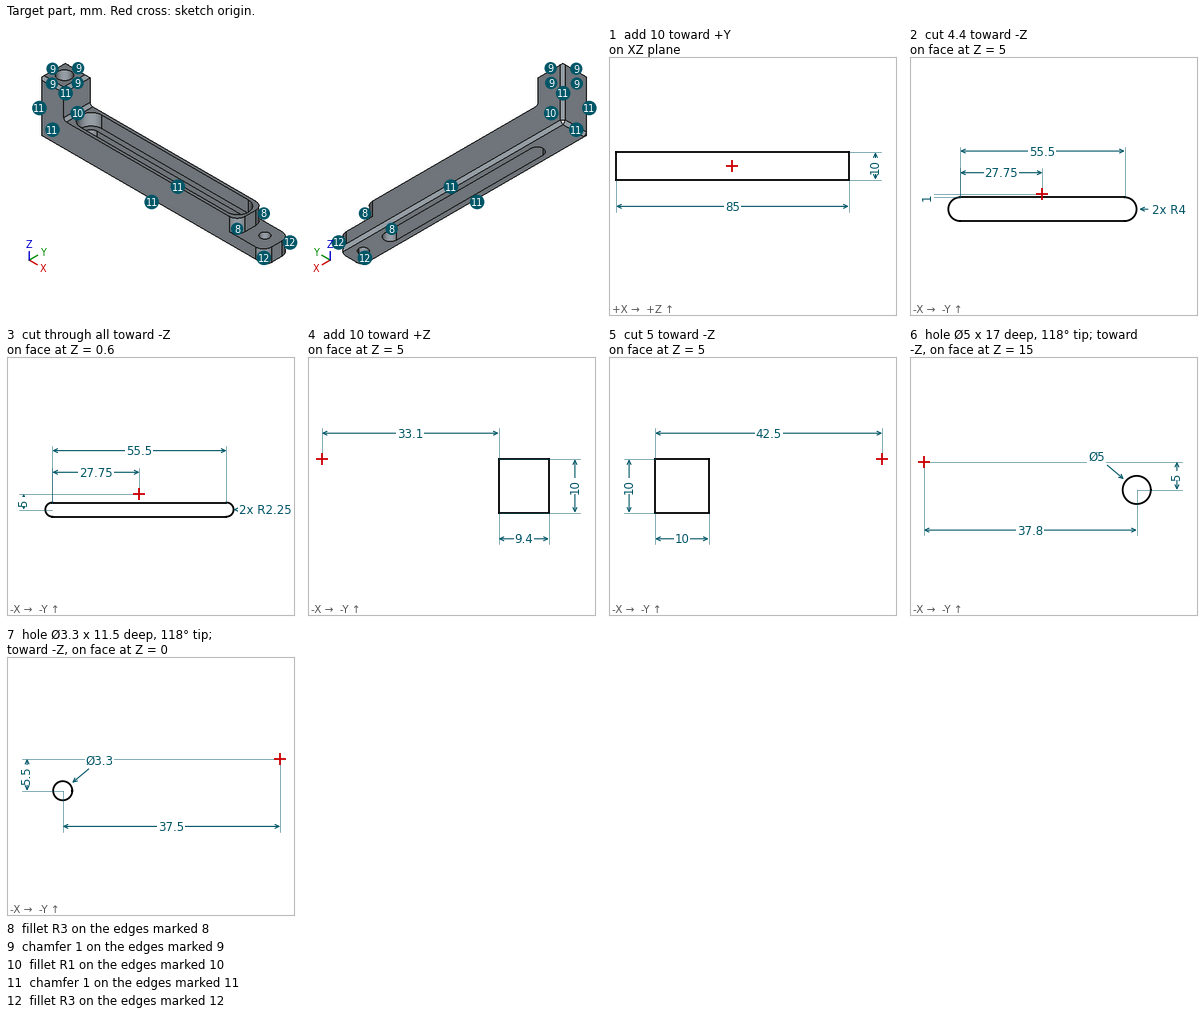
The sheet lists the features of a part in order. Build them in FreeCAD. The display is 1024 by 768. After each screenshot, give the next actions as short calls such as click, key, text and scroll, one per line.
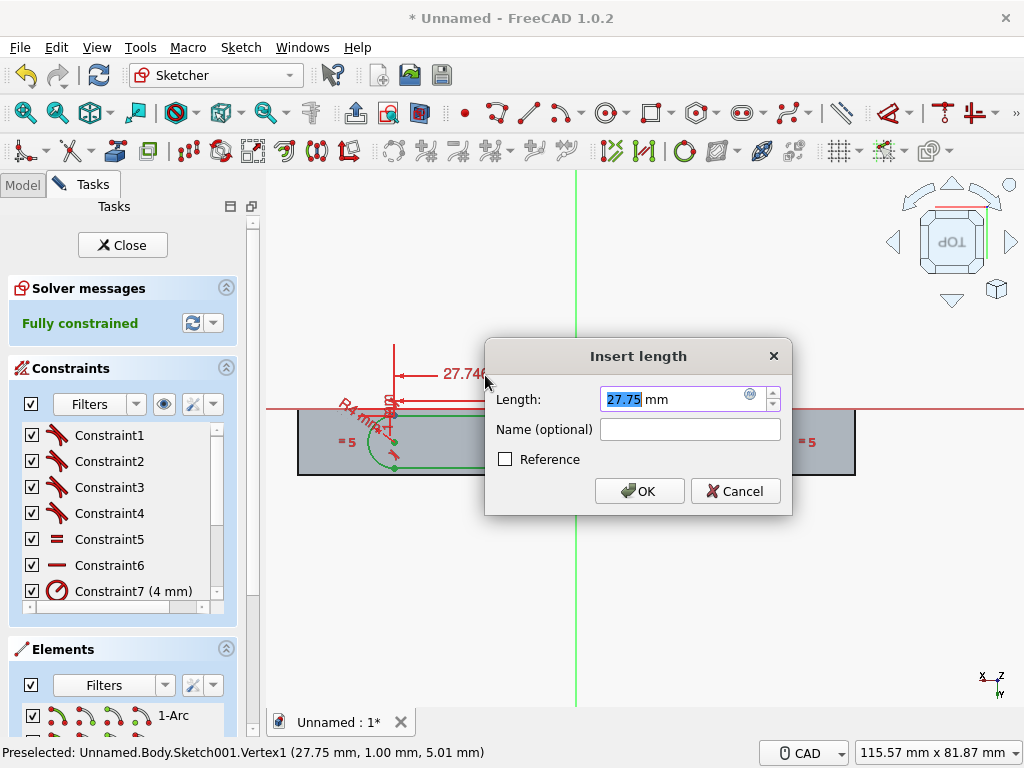
text(27.75)
key(Return)
key(Escape)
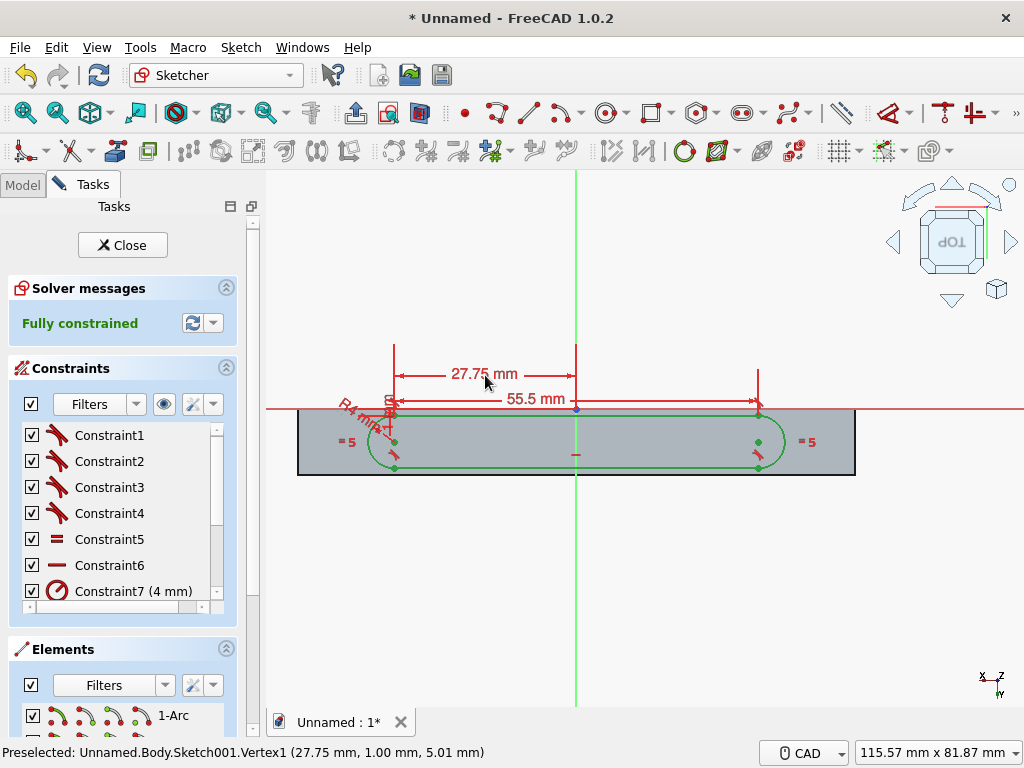
click(123, 245)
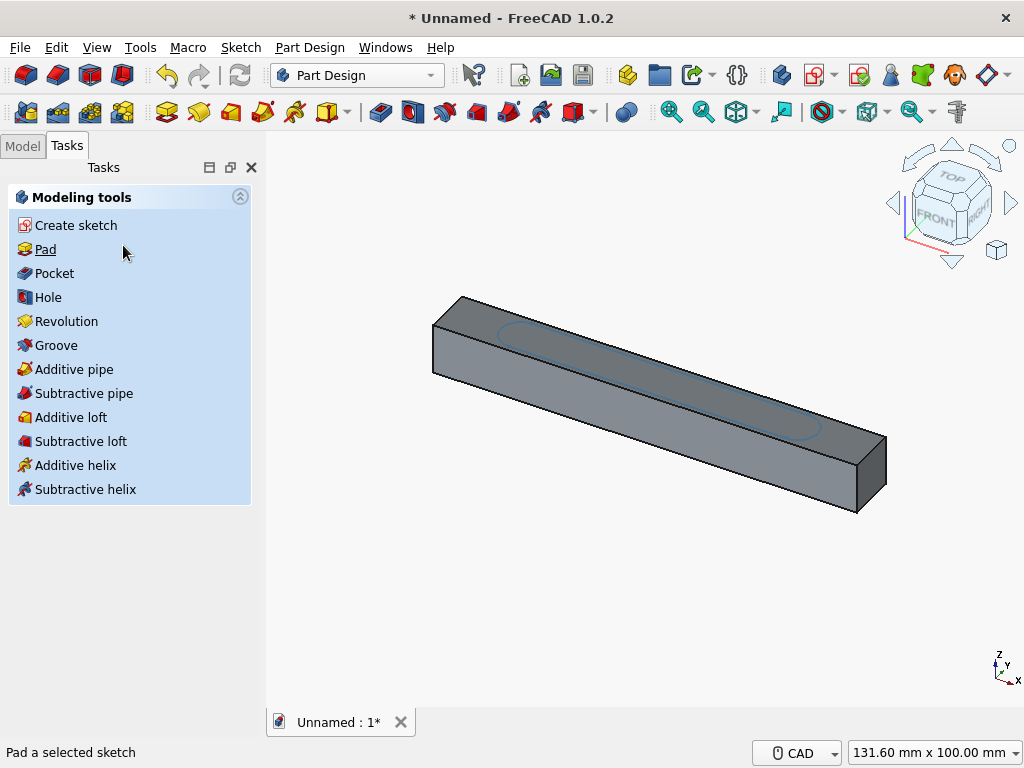
click(382, 112)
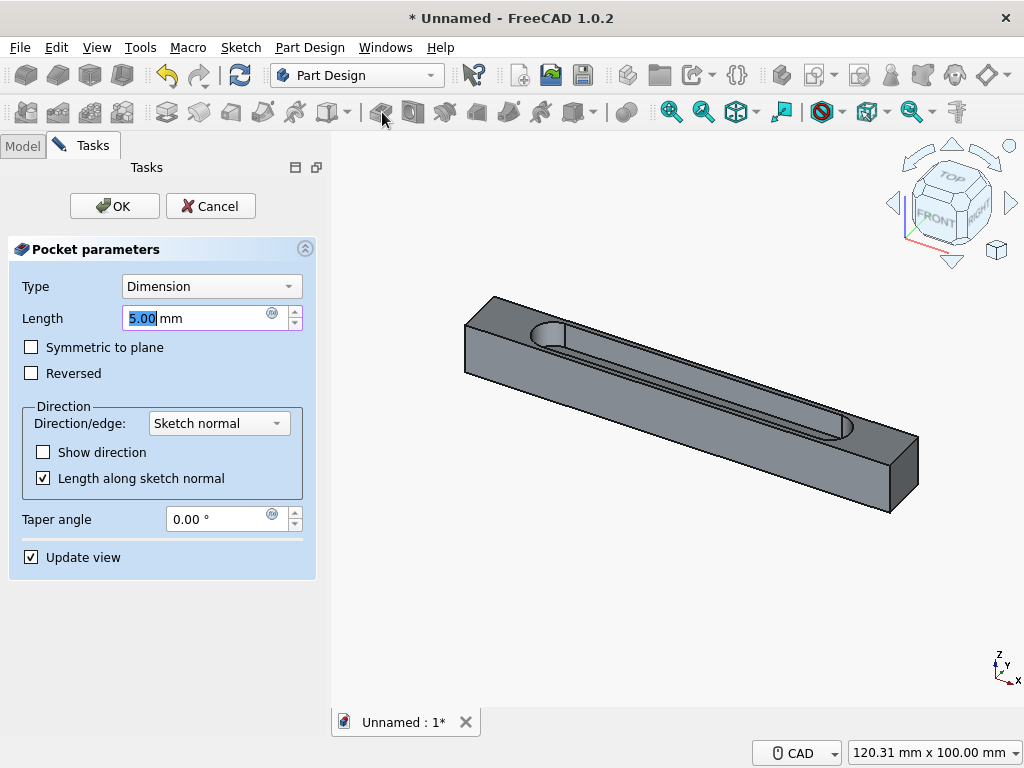
text(4.4)
key(Tab)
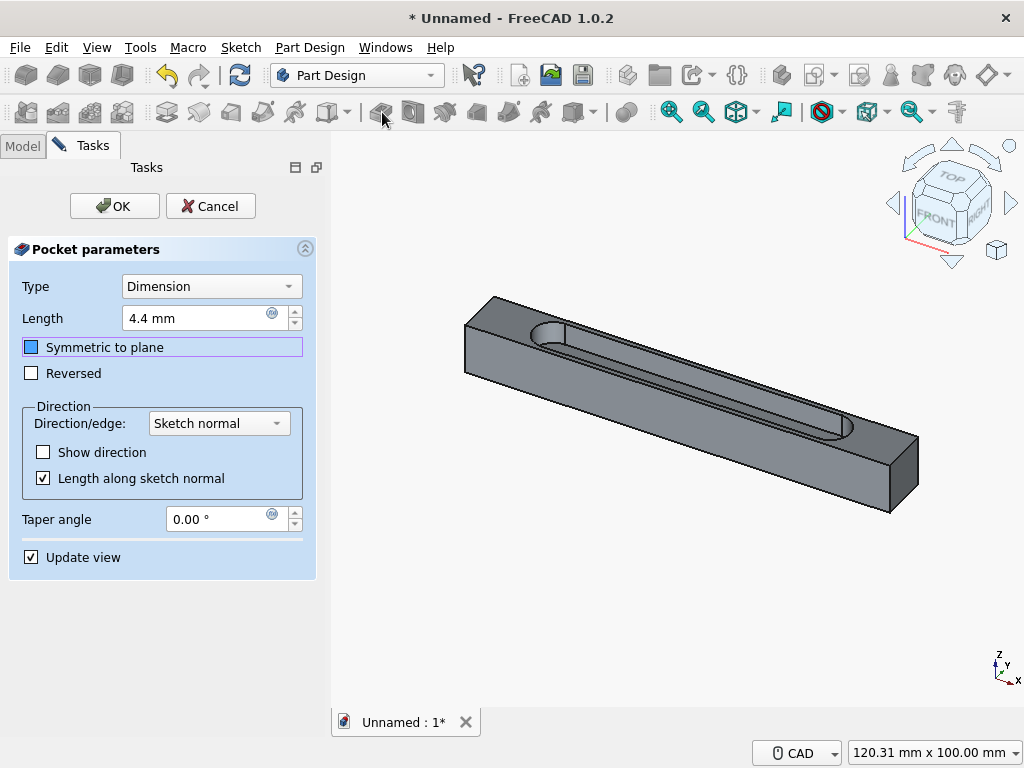
click(115, 206)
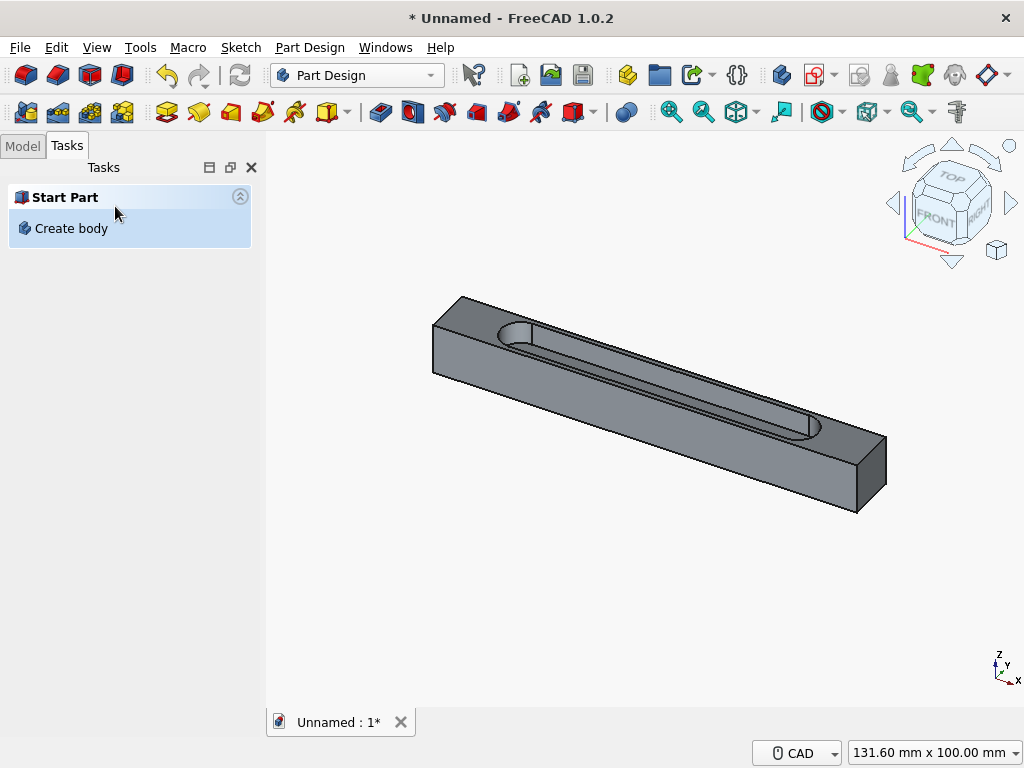
key(0)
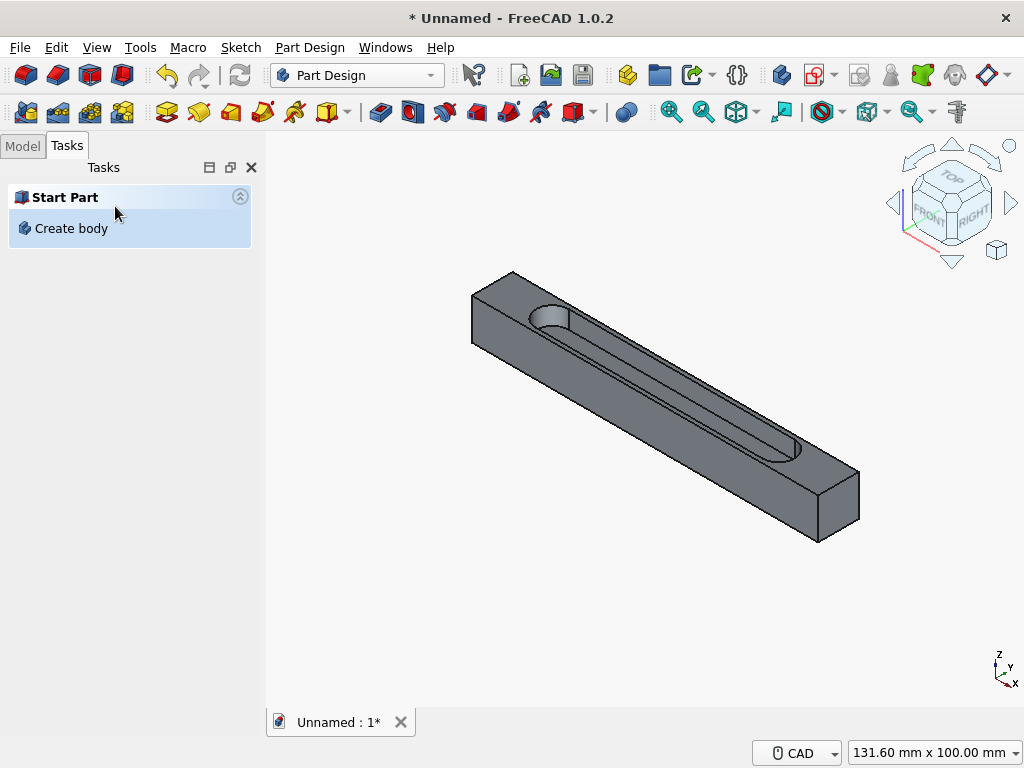
key(2)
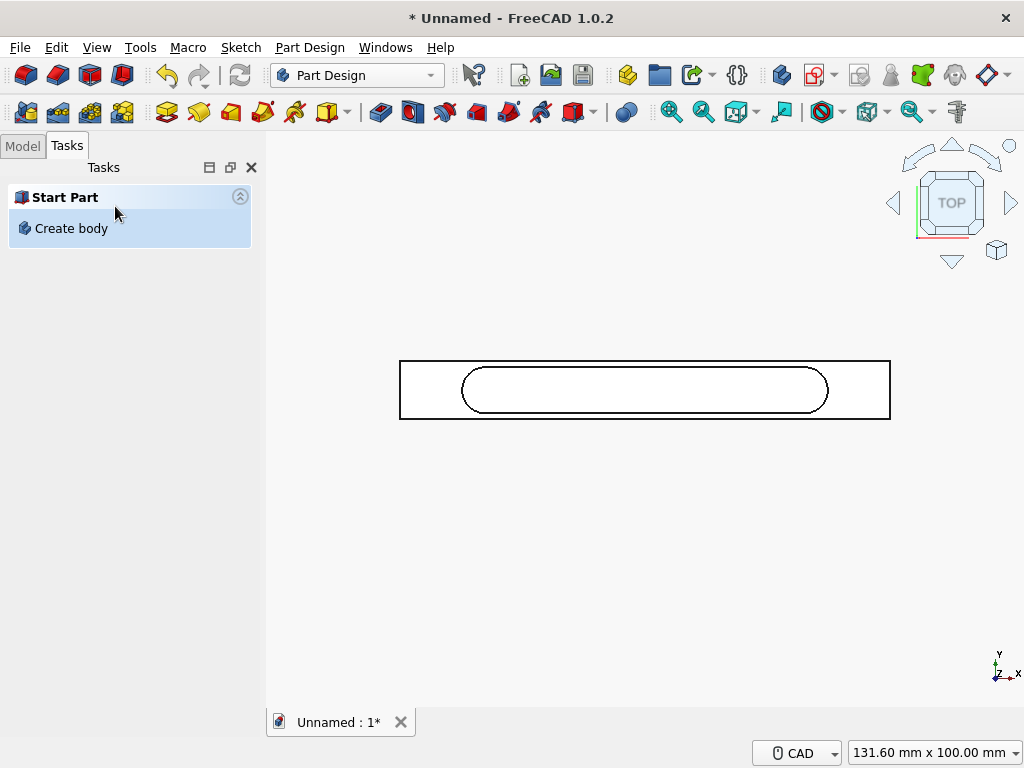
click(802, 389)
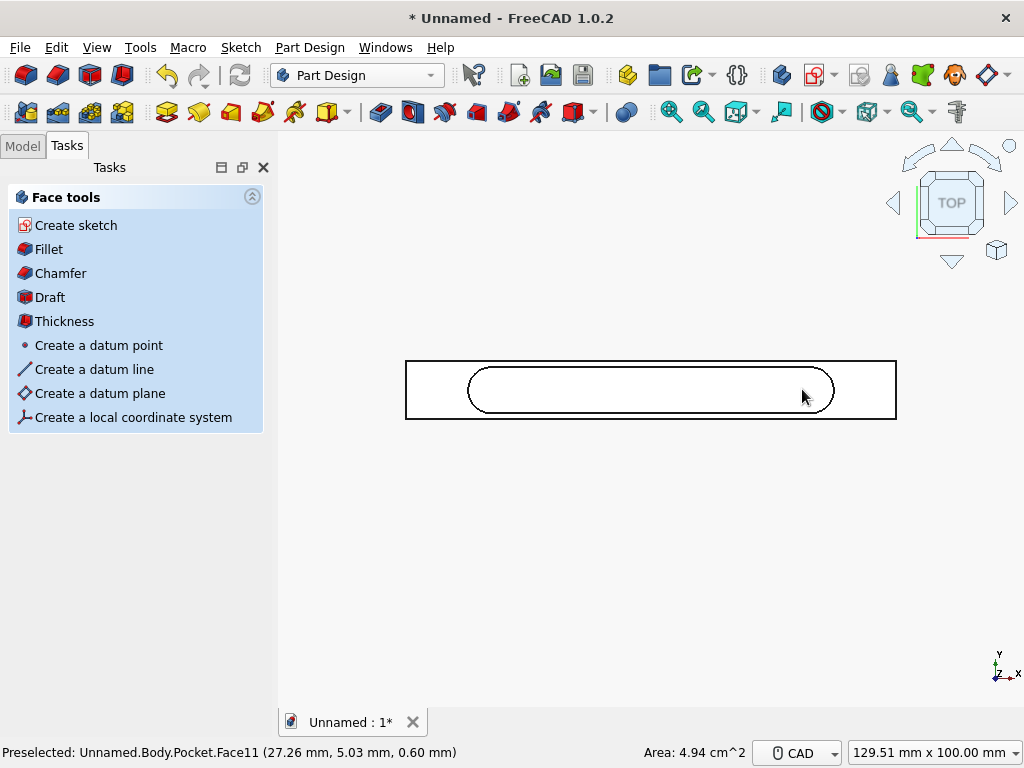
click(814, 76)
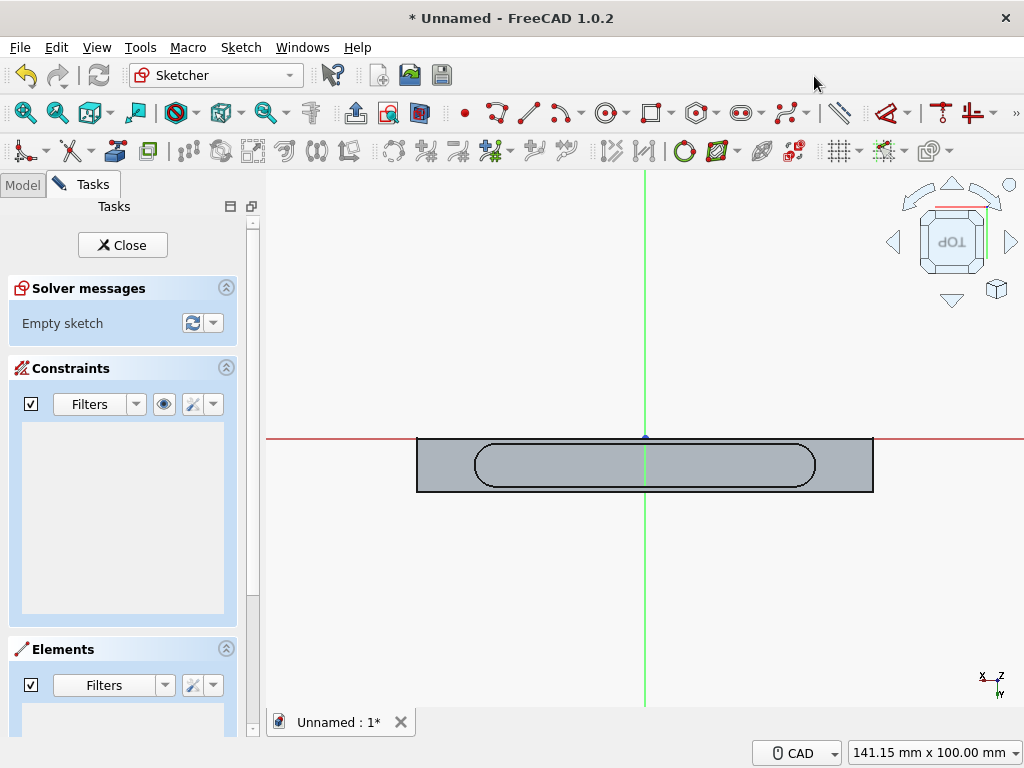
key(q)
key(s)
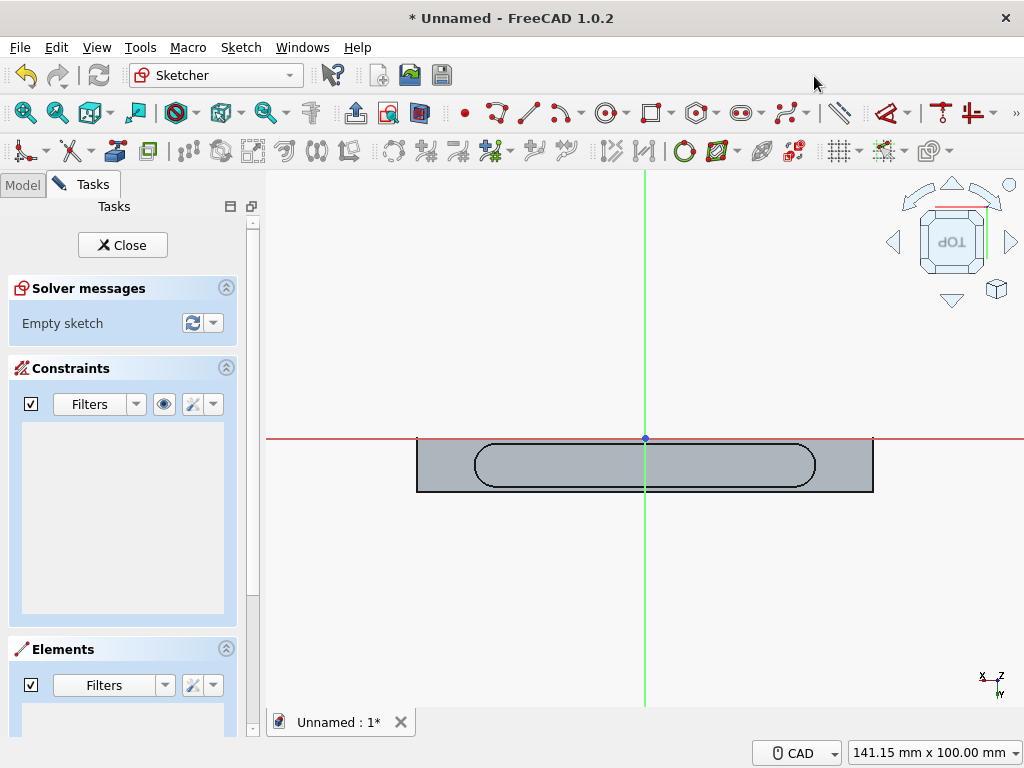
key(g)
key(s)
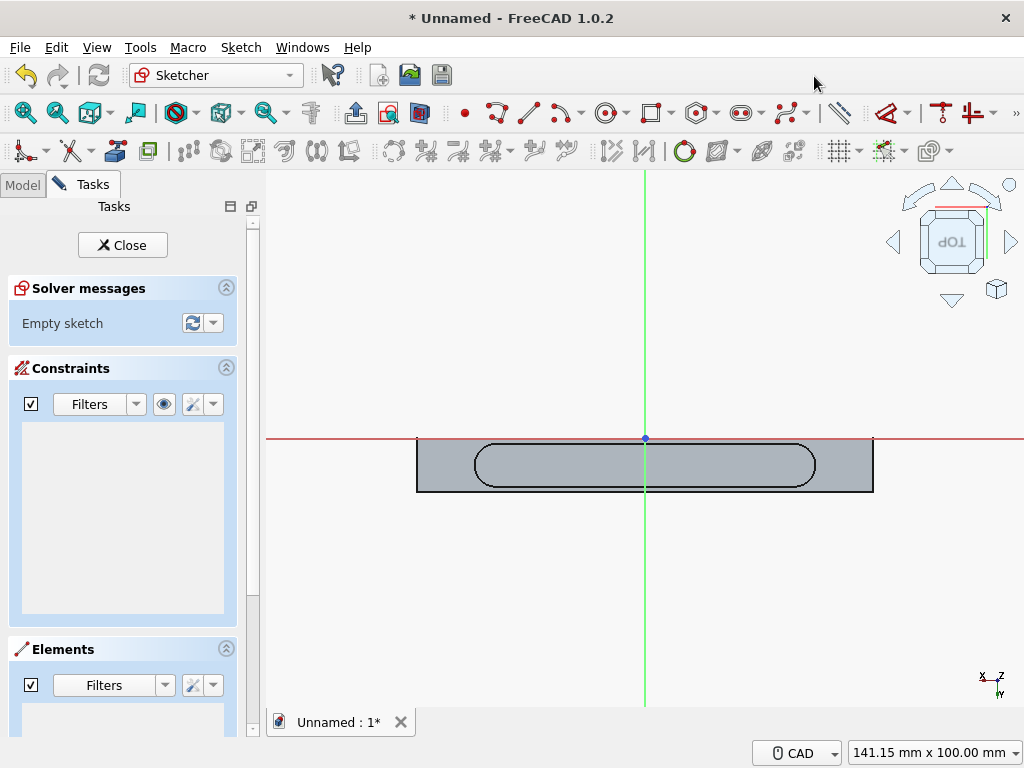
scroll(496, 465, up, 4)